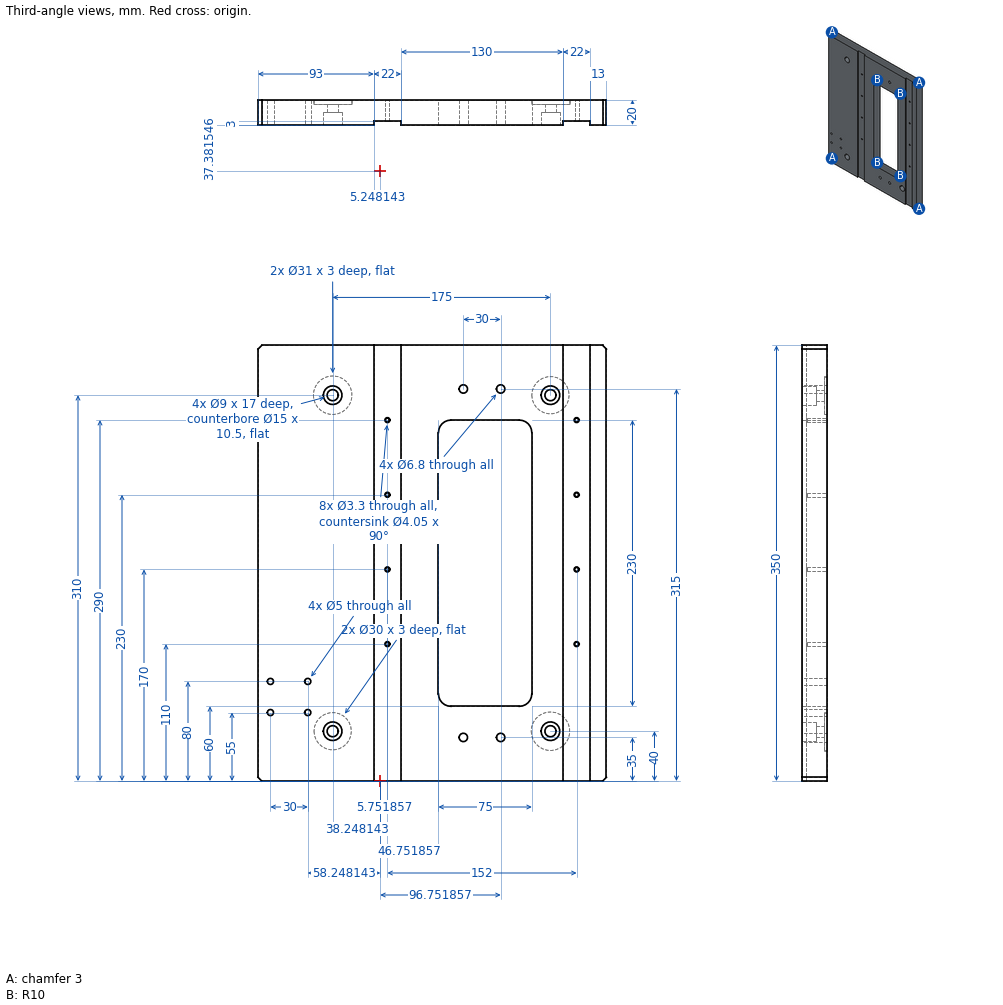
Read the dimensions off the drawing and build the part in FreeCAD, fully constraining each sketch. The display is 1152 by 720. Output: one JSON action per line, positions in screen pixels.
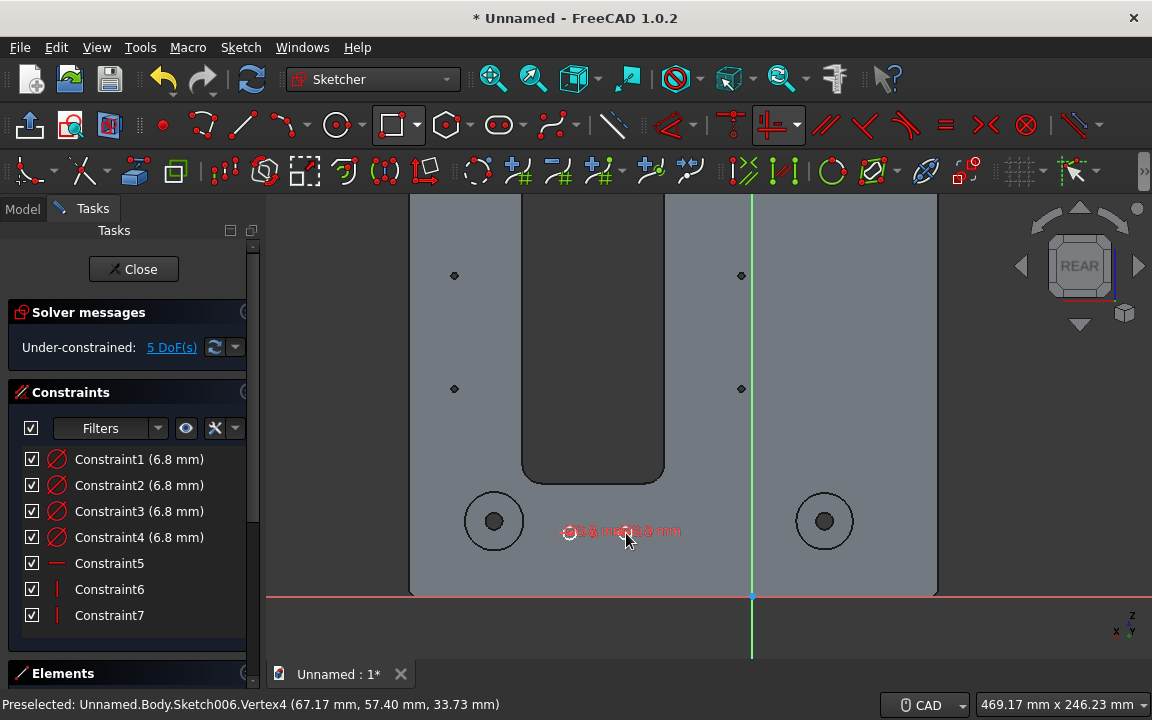
{"action": "left_click", "coordinate": [800, 126]}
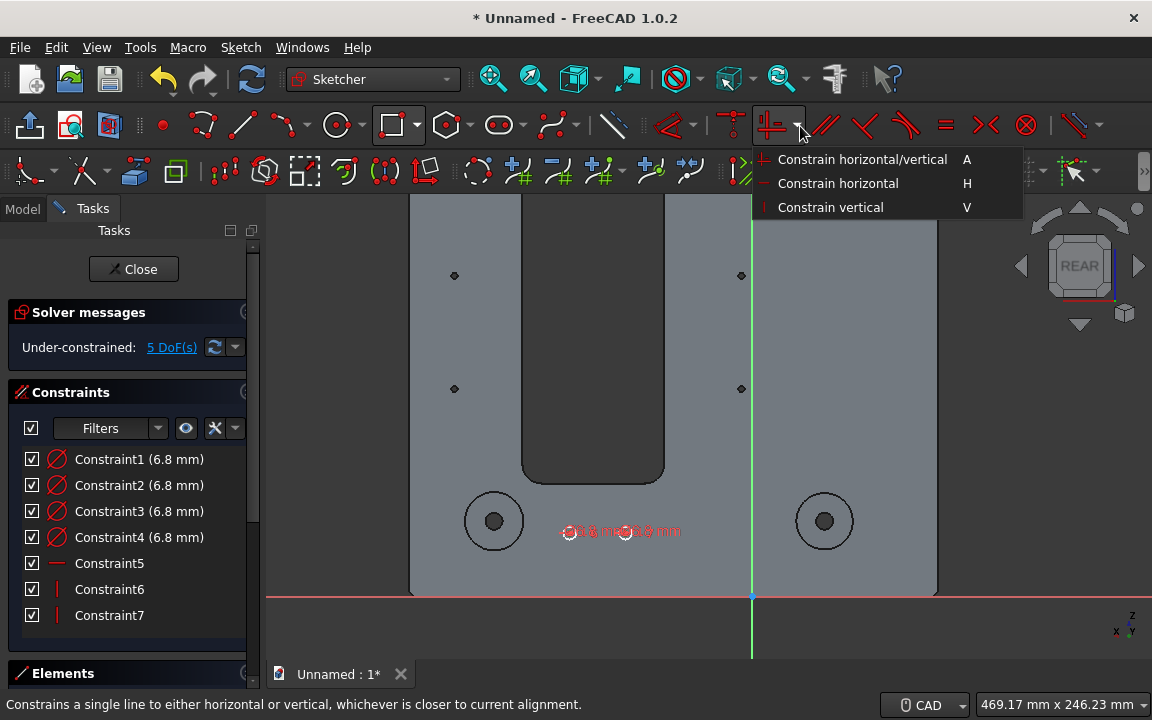
{"action": "left_click", "coordinate": [888, 183]}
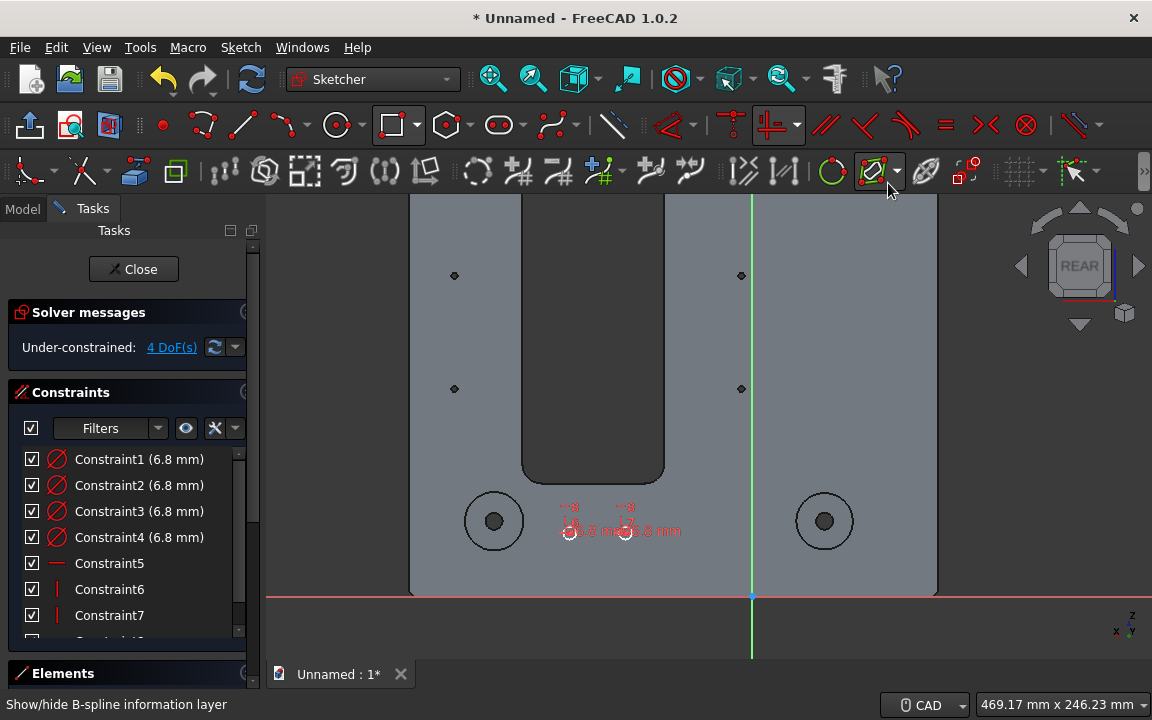
{"action": "left_click", "coordinate": [668, 126]}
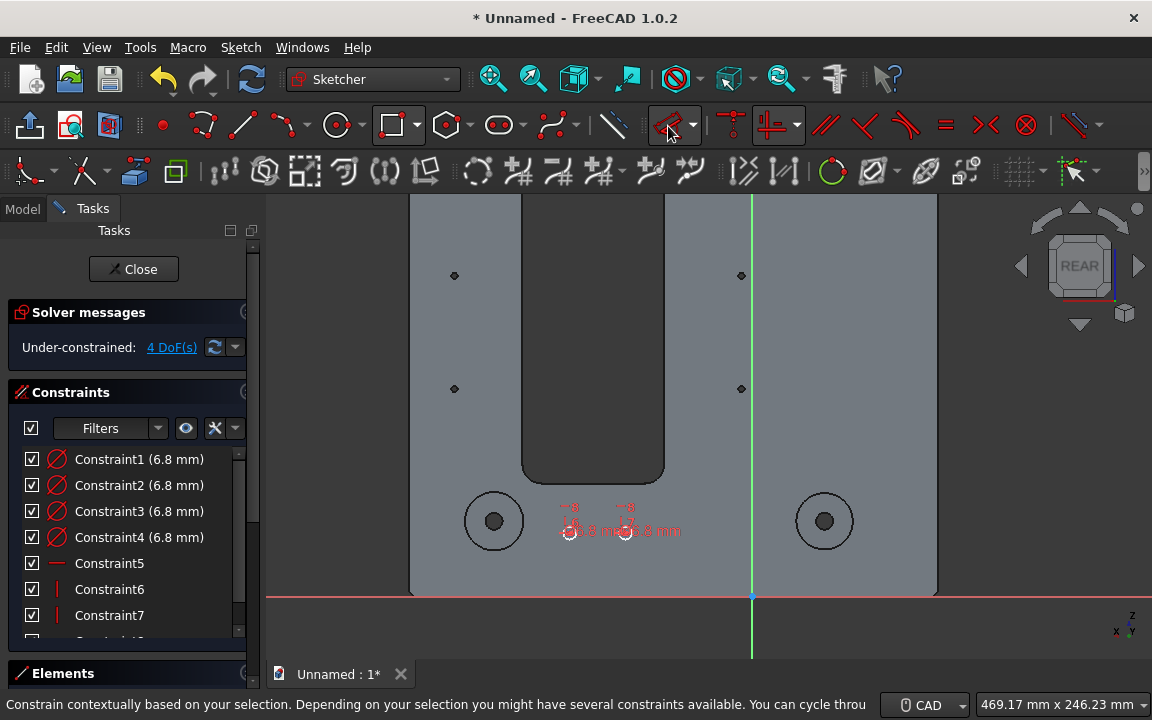
{"action": "left_click", "coordinate": [570, 533]}
{"action": "left_click", "coordinate": [786, 565]}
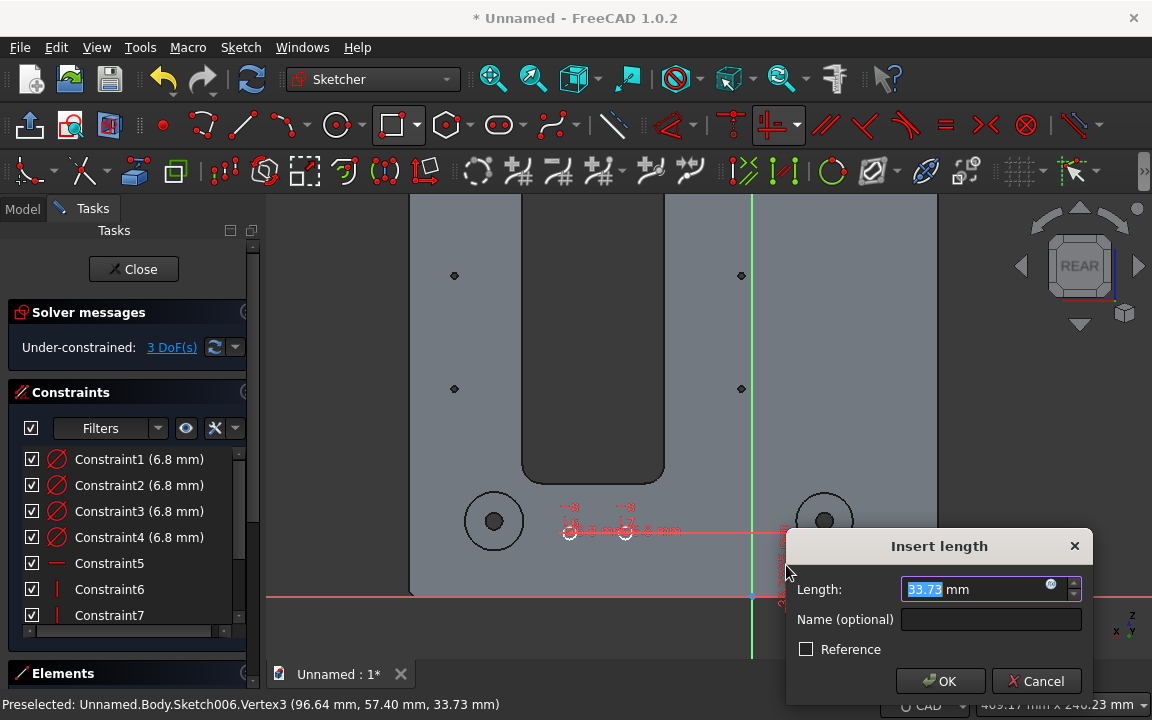
{"action": "type", "text": "35"}
{"action": "key", "text": "Return"}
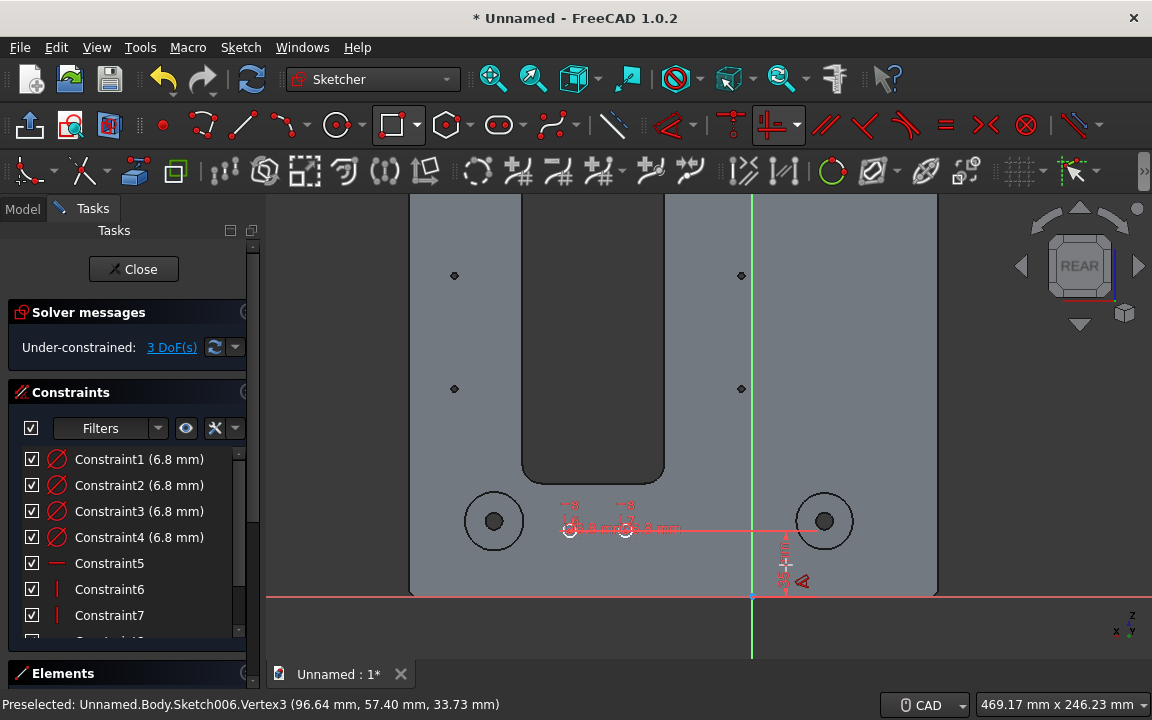
{"action": "scroll", "coordinate": [626, 533], "scroll_direction": "down", "scroll_amount": 4}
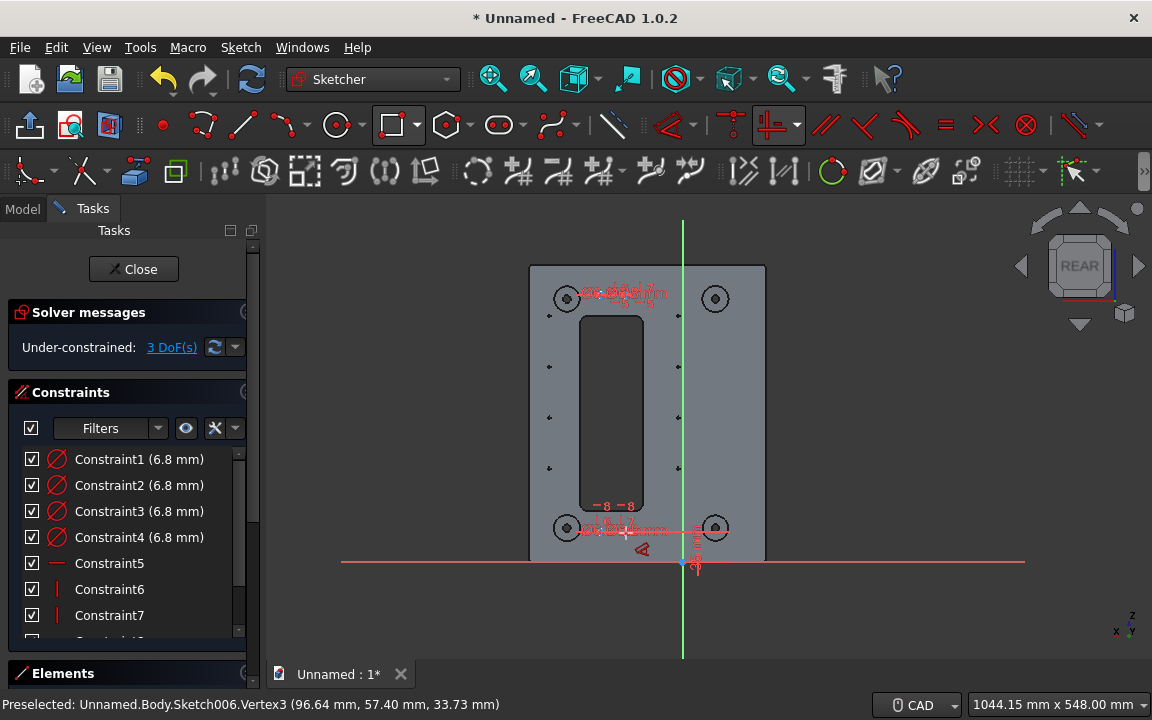
{"action": "left_click", "coordinate": [601, 295]}
{"action": "left_click", "coordinate": [717, 429]}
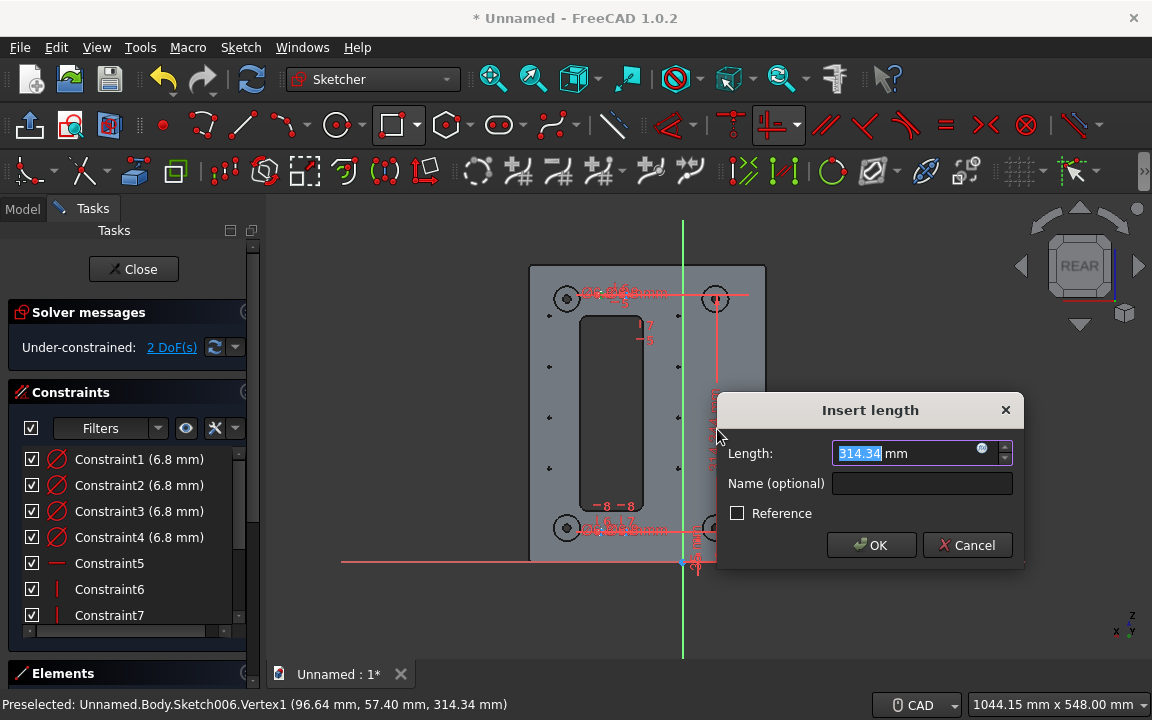
{"action": "type", "text": "315"}
{"action": "key", "text": "Return"}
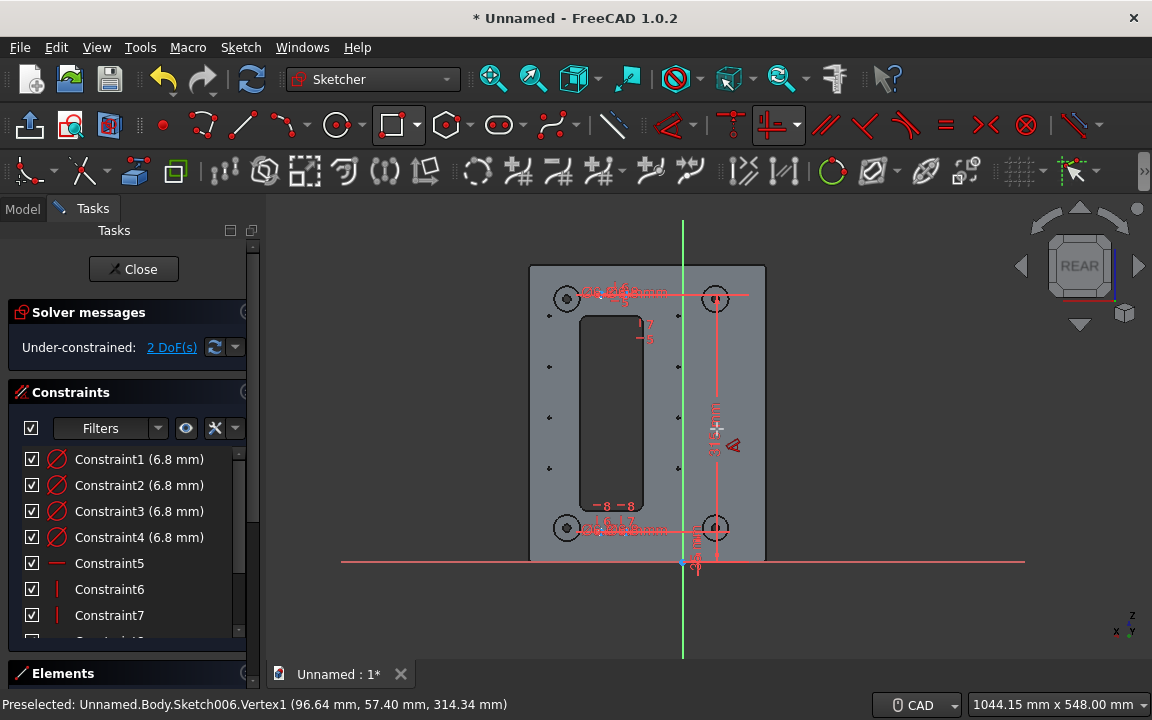
{"action": "scroll", "coordinate": [601, 295], "scroll_direction": "up", "scroll_amount": 3}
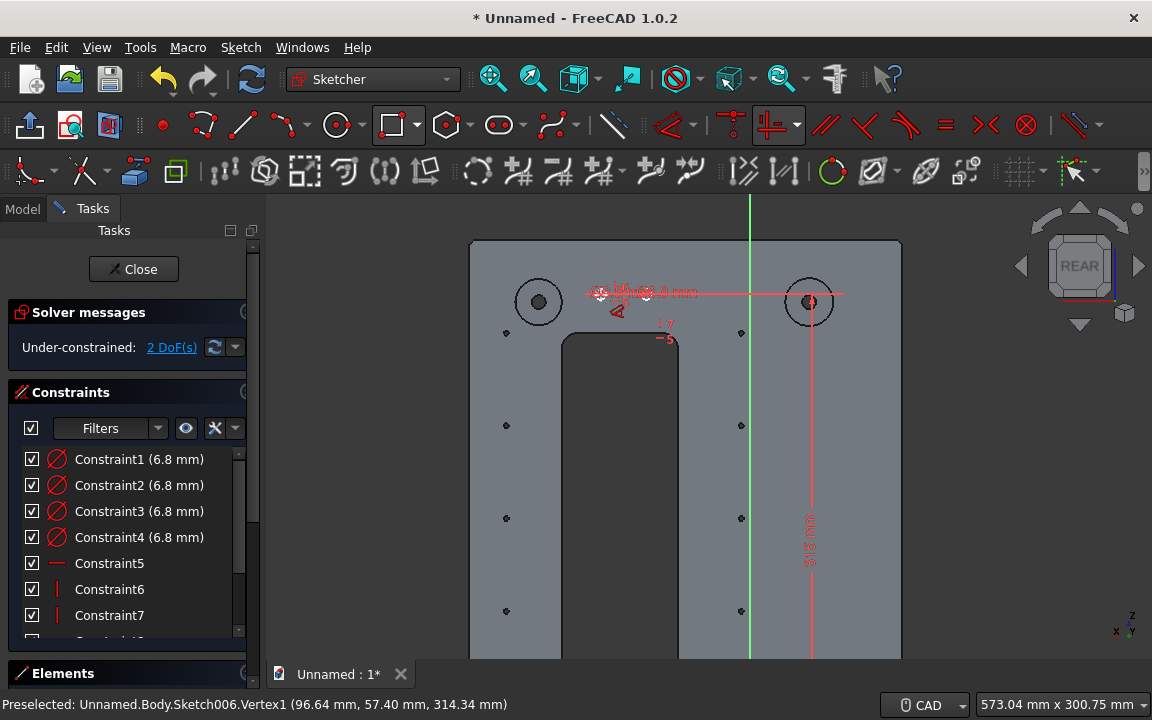
{"action": "left_click", "coordinate": [601, 294]}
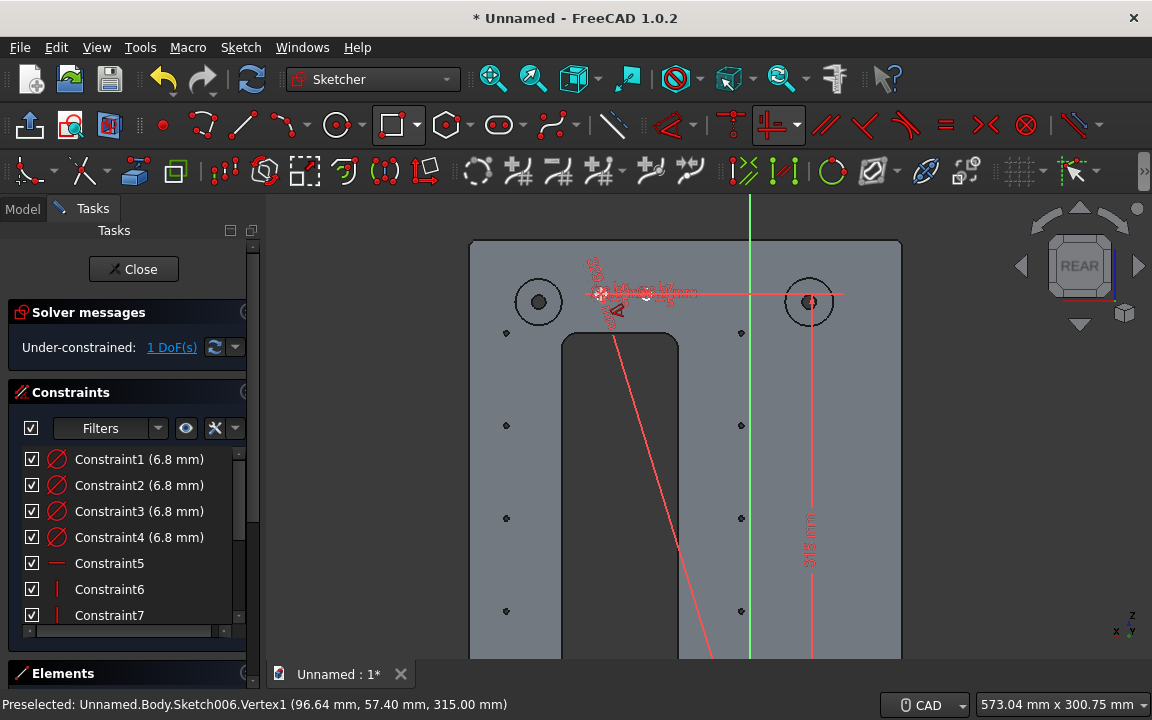
{"action": "left_click", "coordinate": [646, 294]}
{"action": "left_click", "coordinate": [623, 260]}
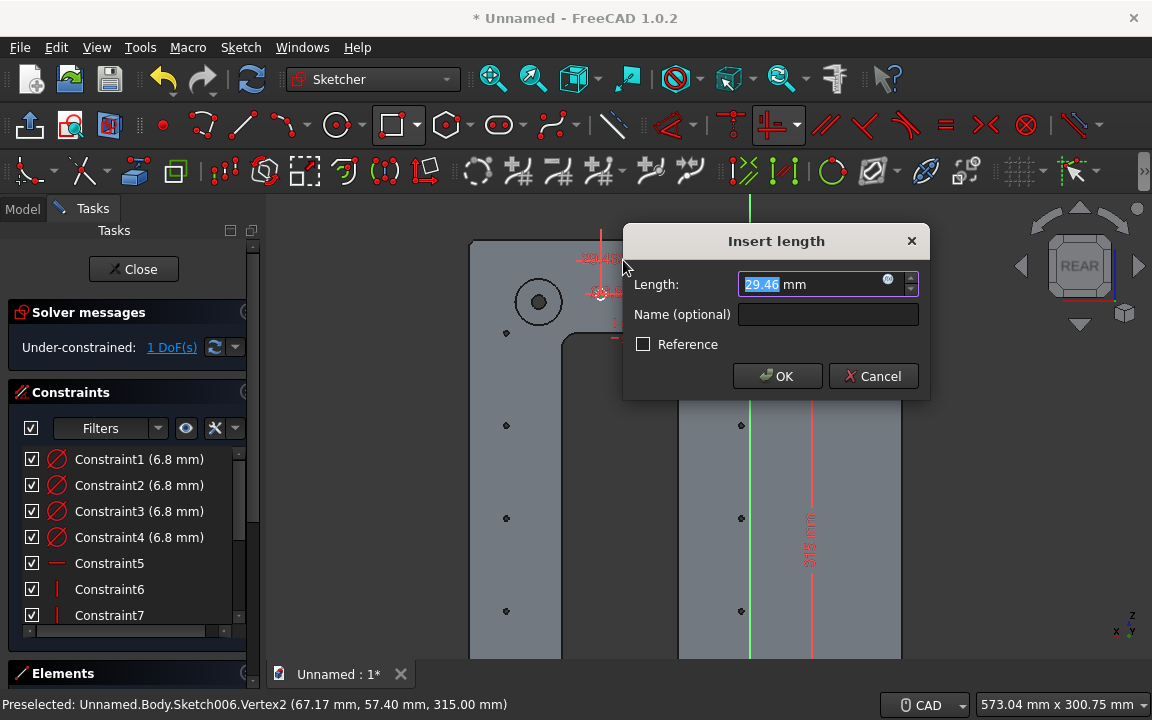
{"action": "type", "text": "30"}
{"action": "key", "text": "Return"}